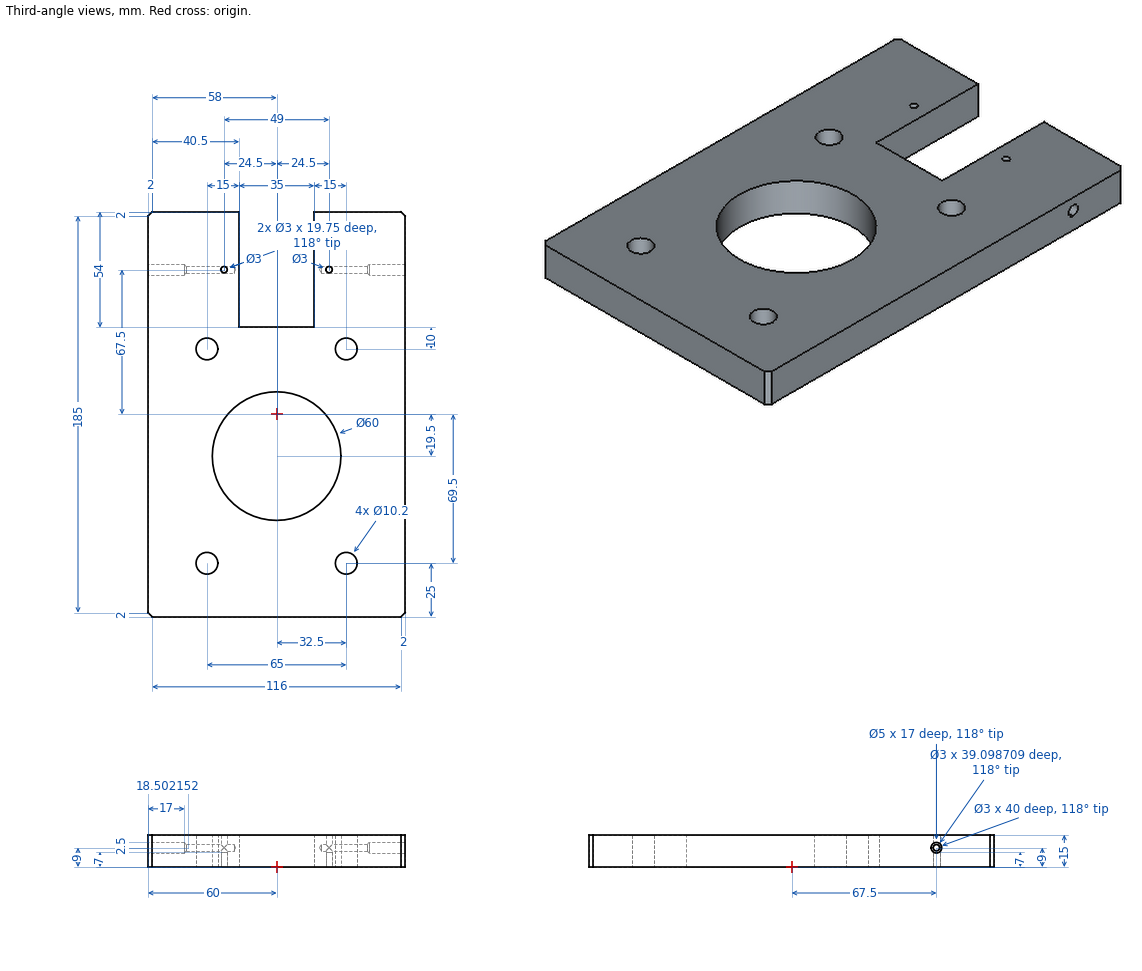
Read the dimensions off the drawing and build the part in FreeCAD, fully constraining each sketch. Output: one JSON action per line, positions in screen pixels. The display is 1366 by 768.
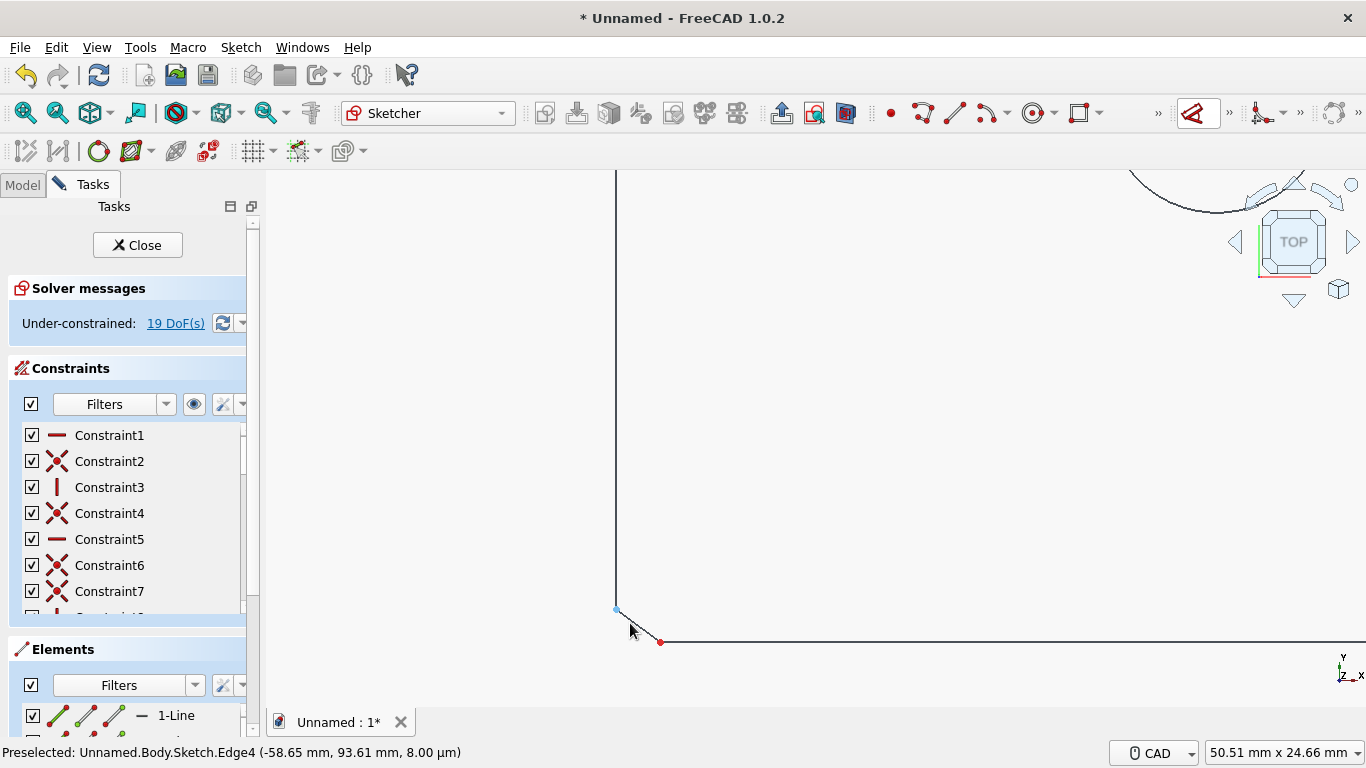
{"action": "left_click", "coordinate": [629, 619]}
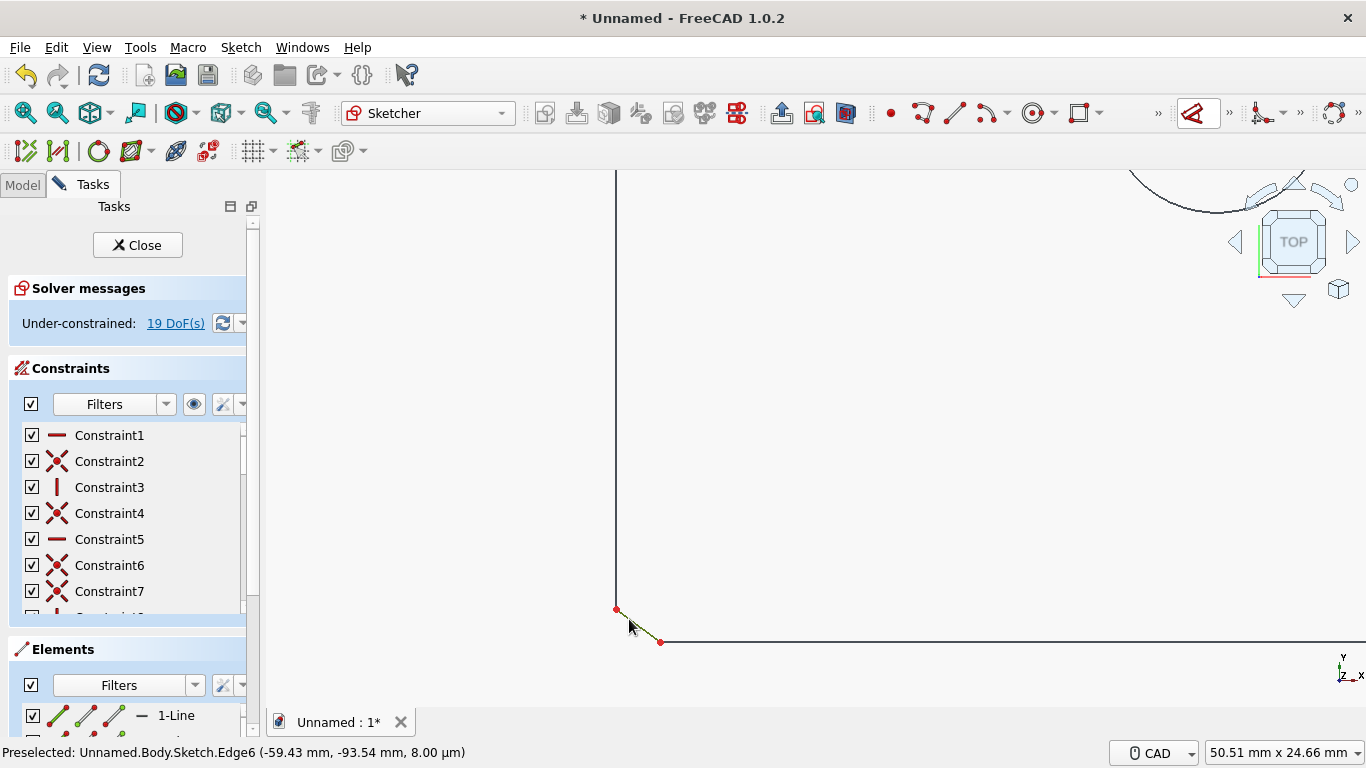
{"action": "key", "text": "l"}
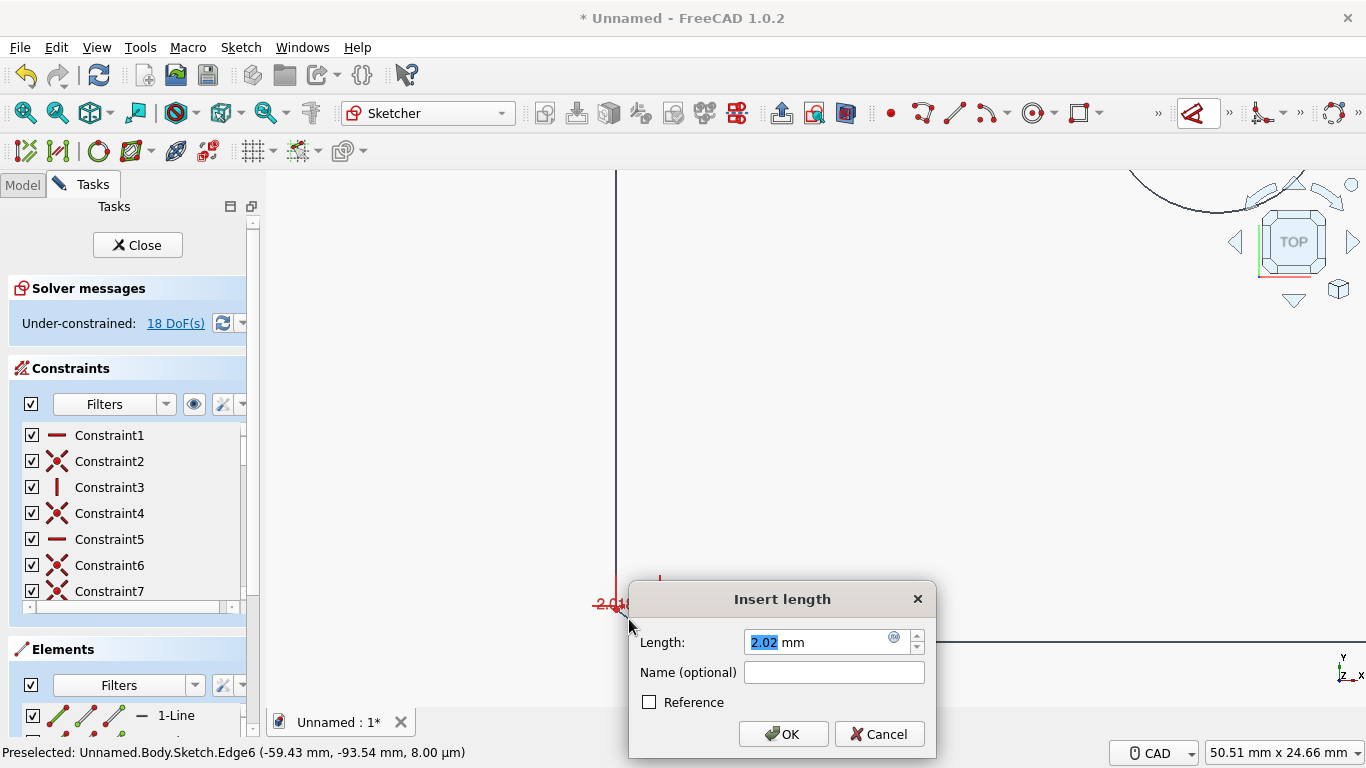
{"action": "type", "text": "2"}
{"action": "key", "text": "Return"}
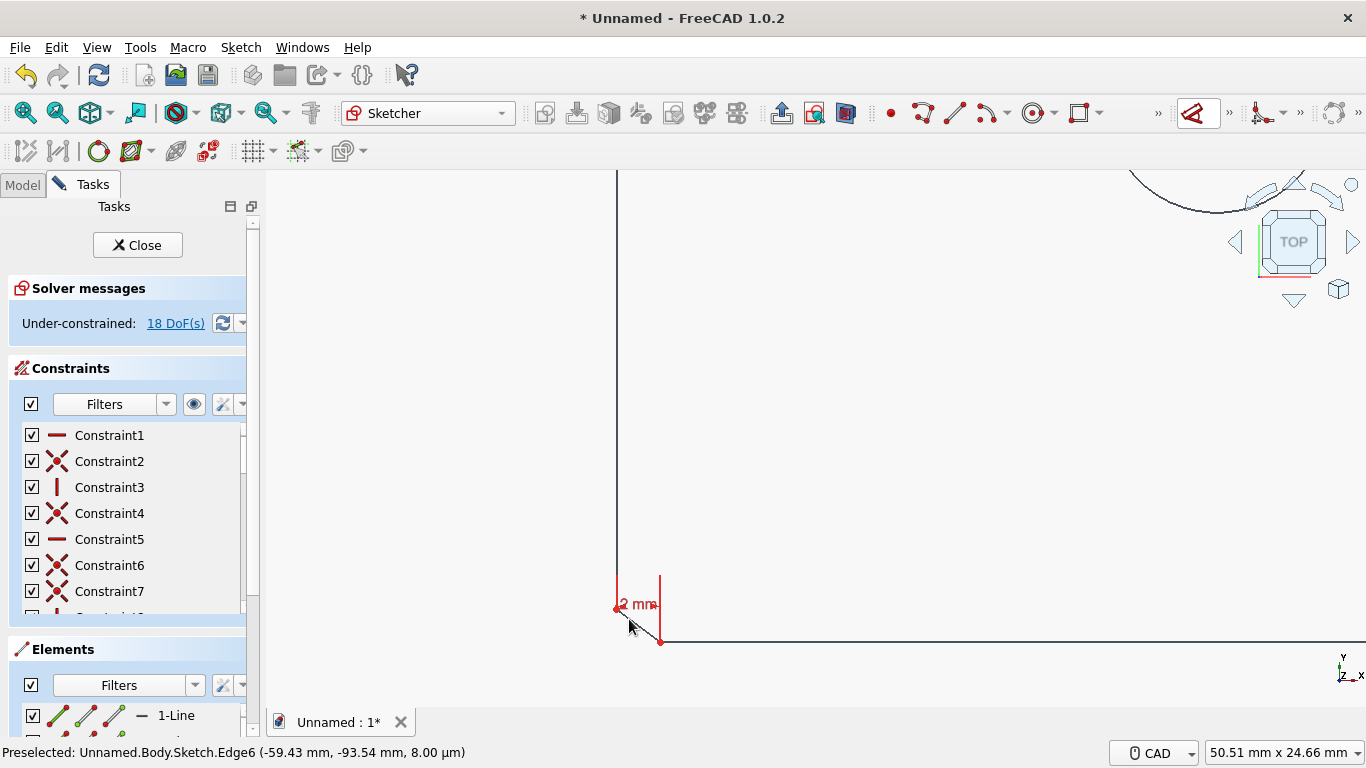
{"action": "left_click", "coordinate": [630, 619]}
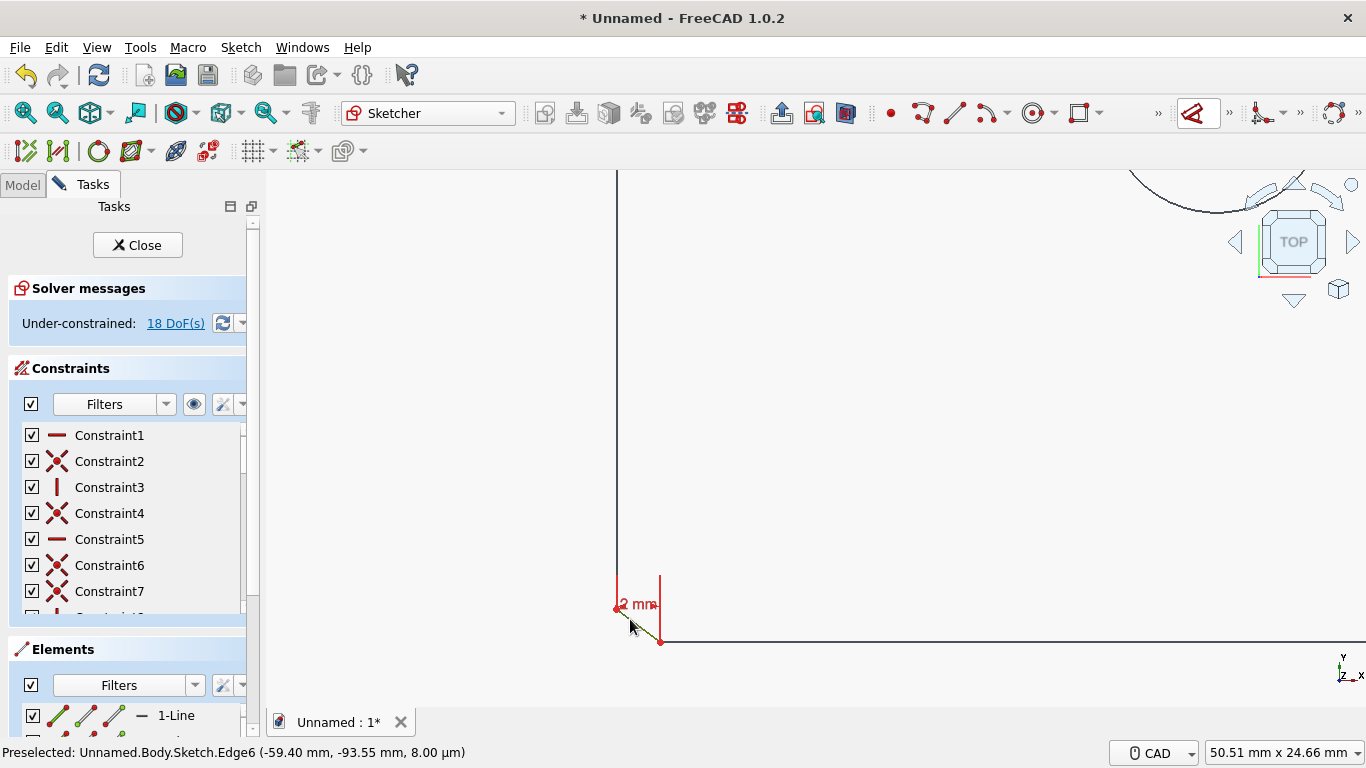
{"action": "key", "text": "i"}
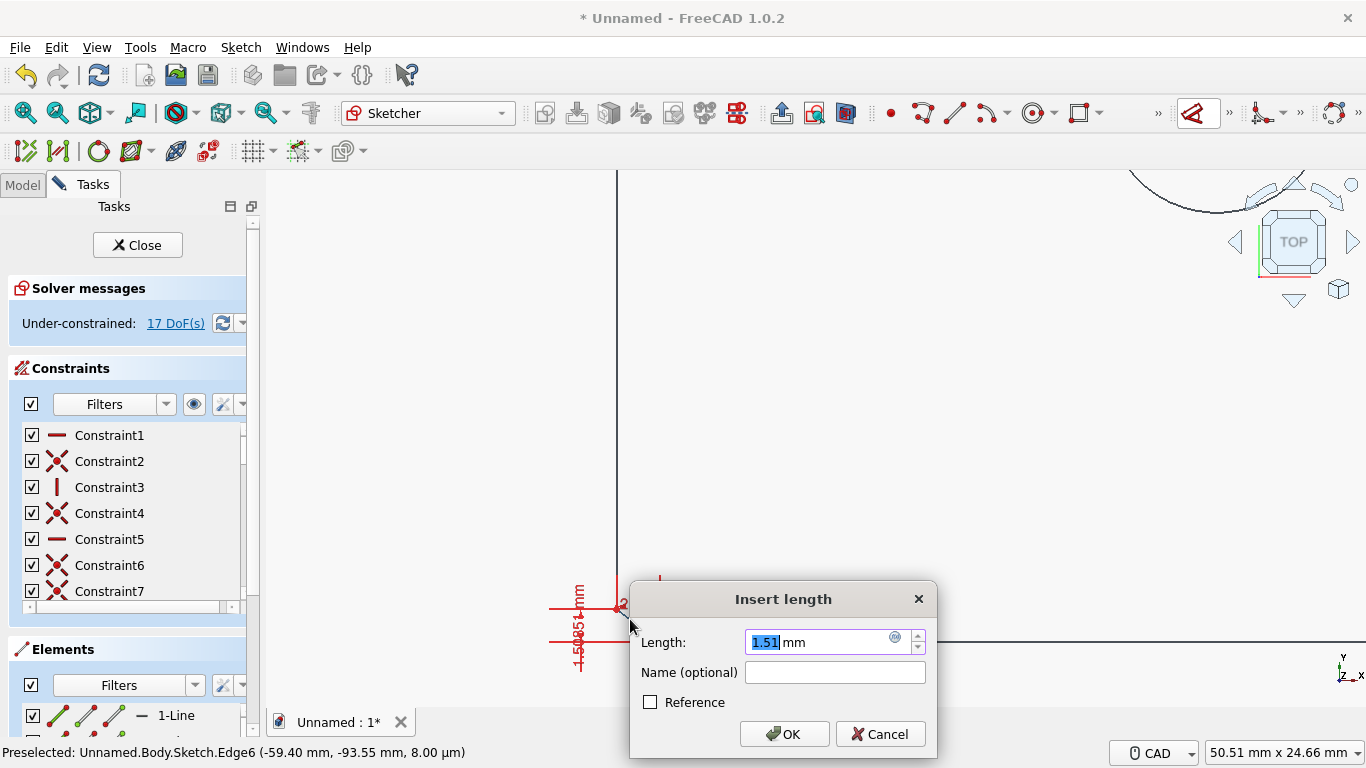
{"action": "type", "text": "2"}
{"action": "key", "text": "Return"}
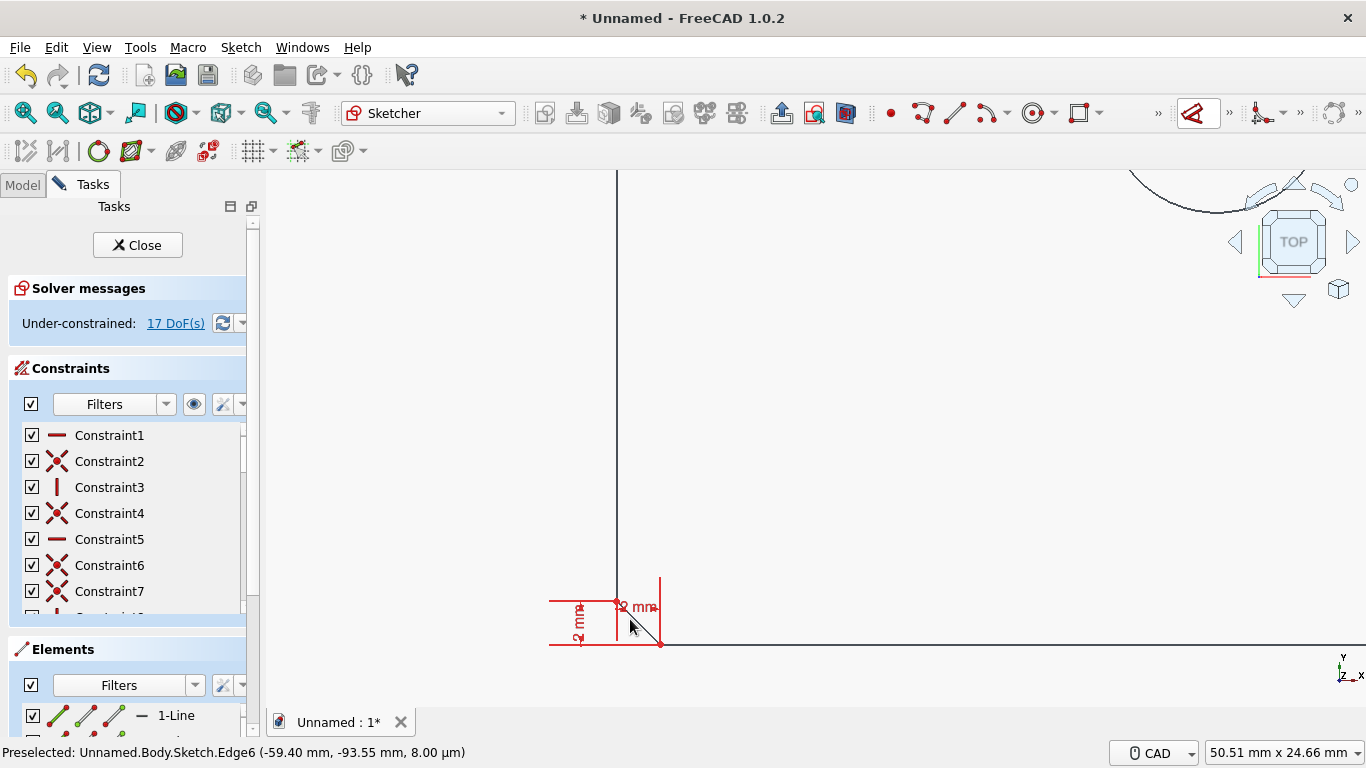
{"action": "scroll", "coordinate": [630, 624], "scroll_direction": "down", "scroll_amount": 12}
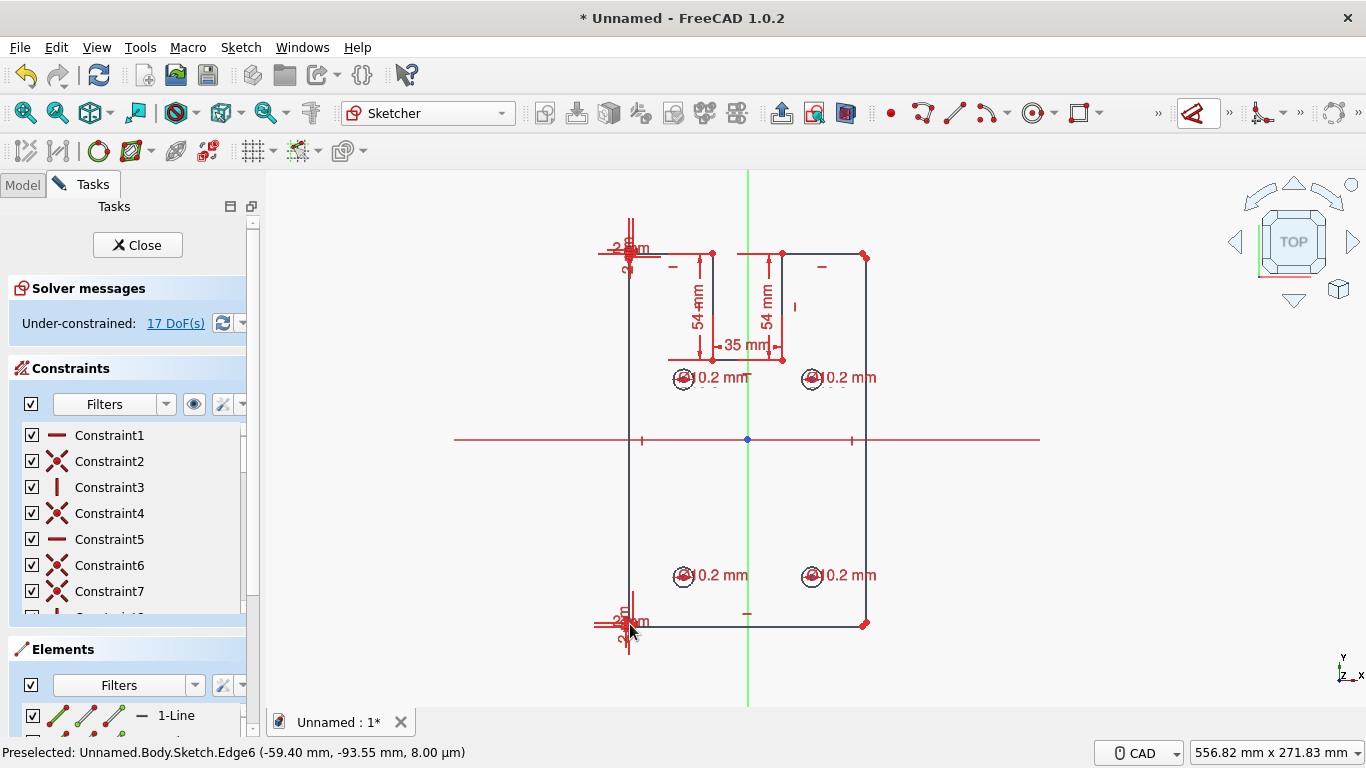
{"action": "scroll", "coordinate": [863, 625], "scroll_direction": "up", "scroll_amount": 12}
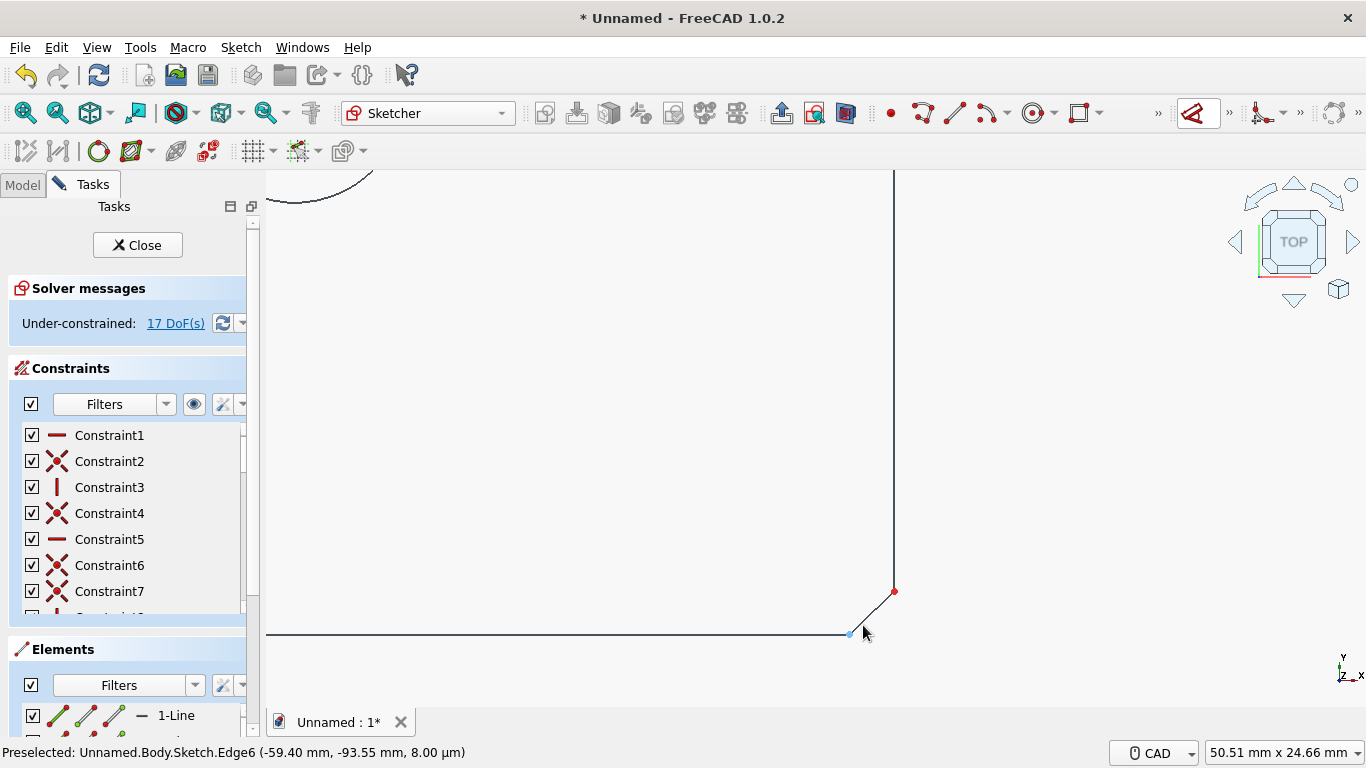
{"action": "left_click", "coordinate": [863, 622]}